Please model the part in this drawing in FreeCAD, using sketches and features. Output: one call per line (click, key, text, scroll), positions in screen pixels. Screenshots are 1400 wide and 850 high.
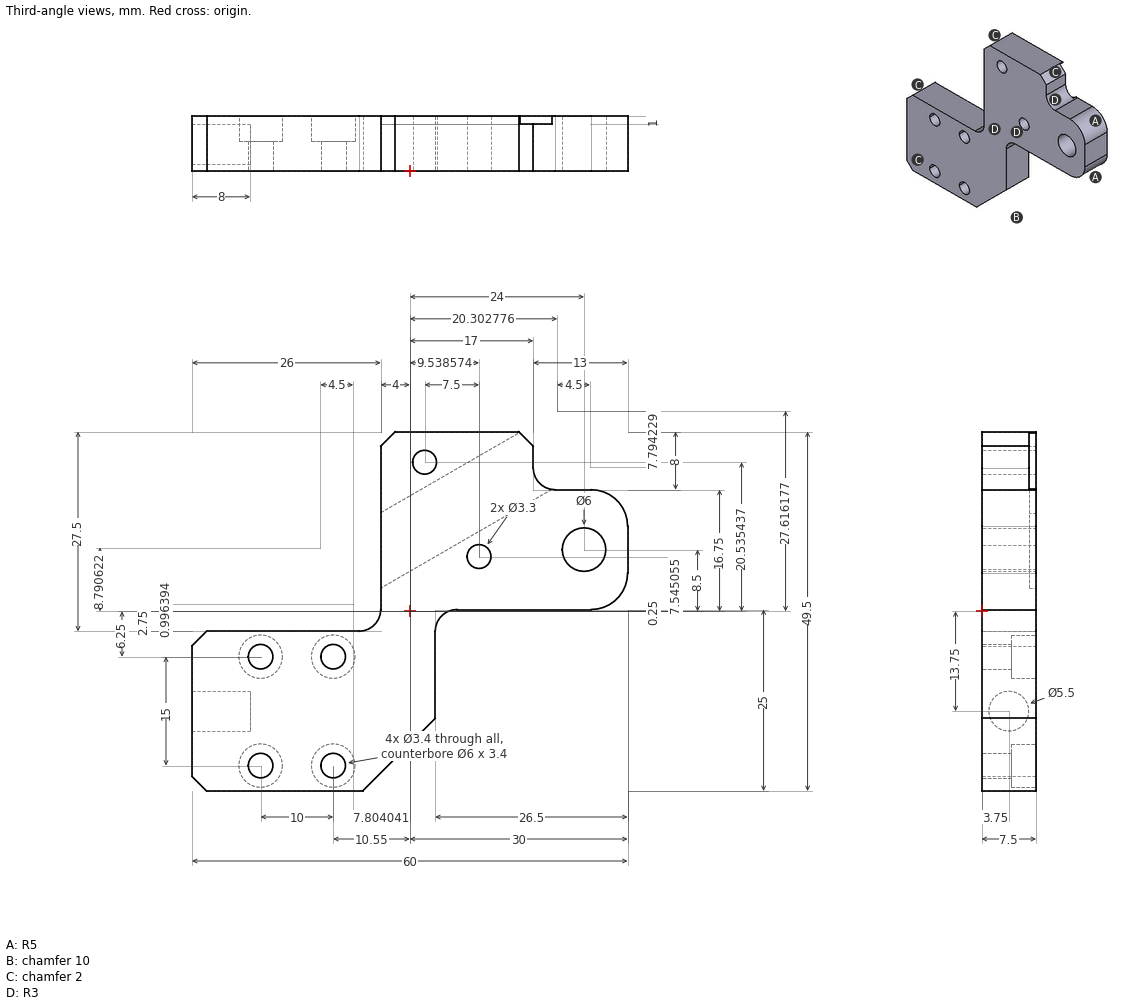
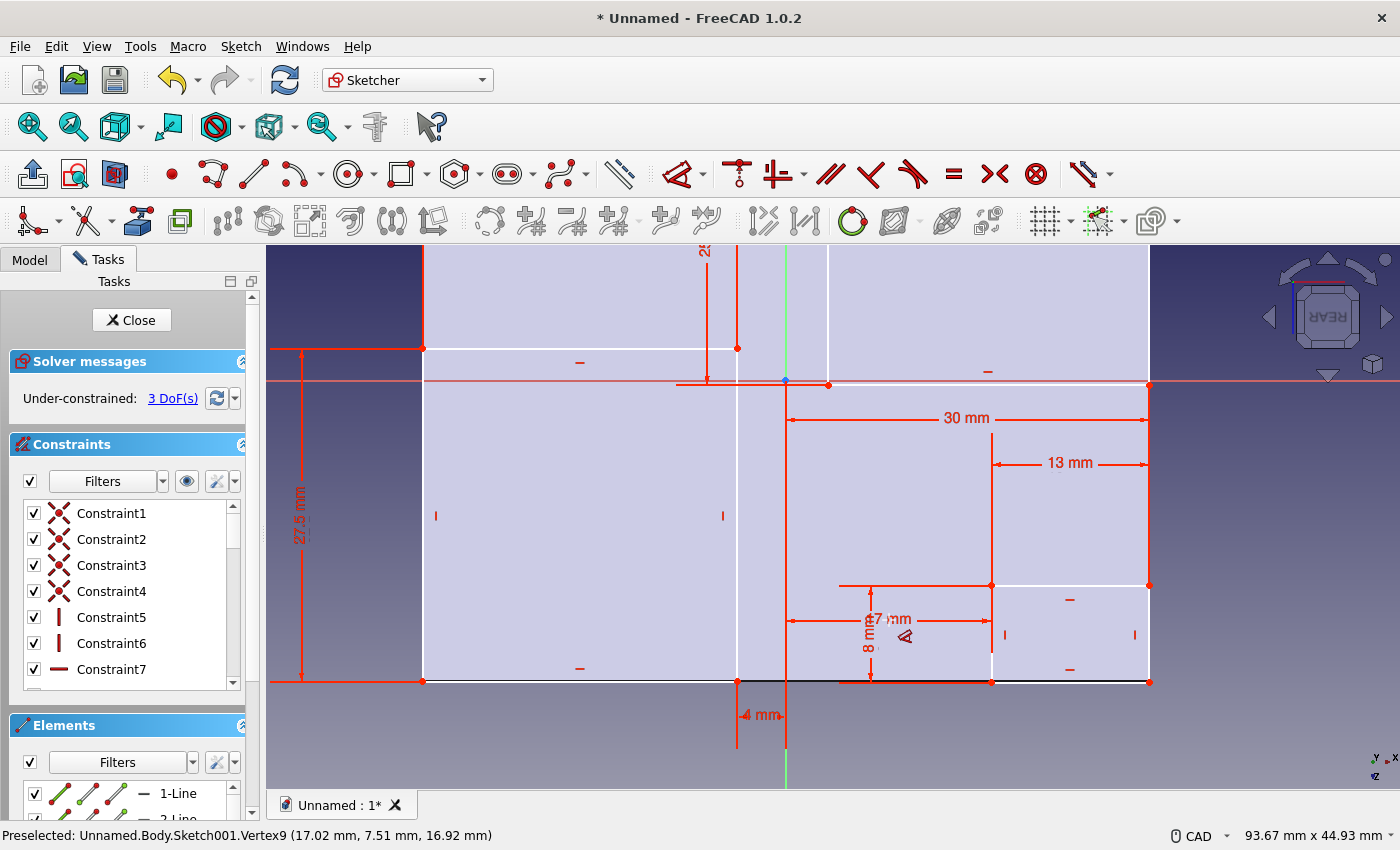
scroll(828, 385, up, 13)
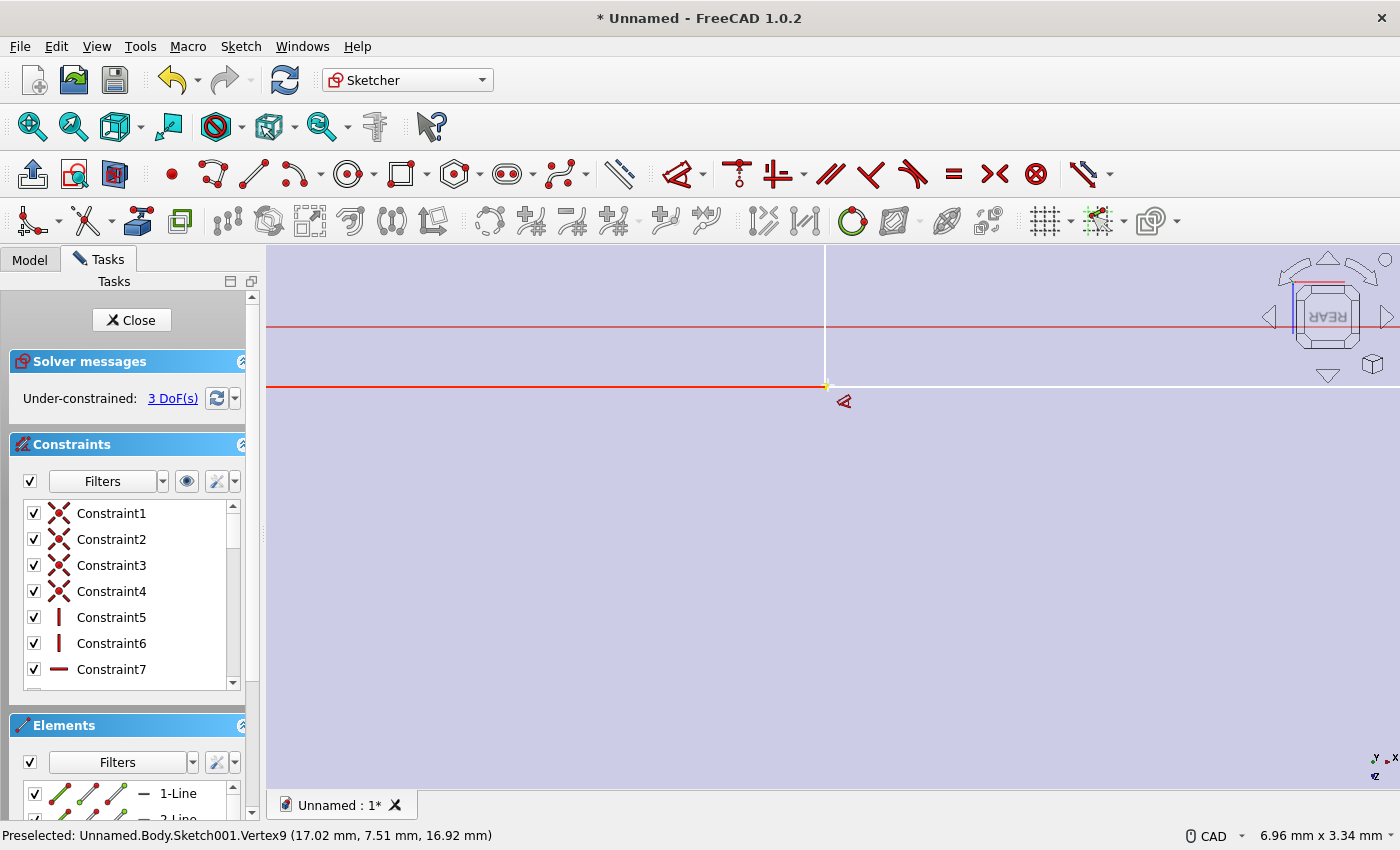
click(825, 387)
click(859, 357)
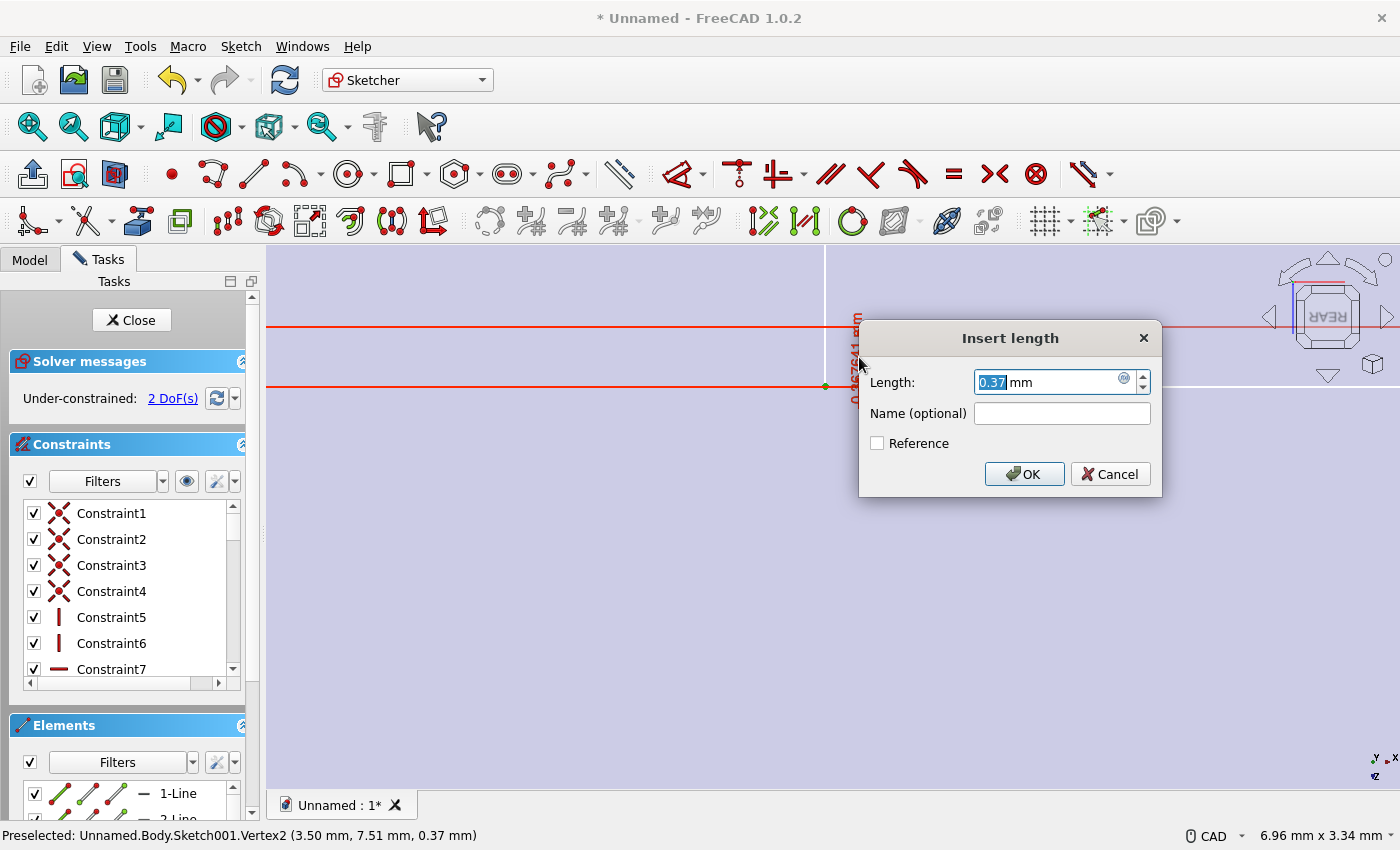
text(0.25)
key(Return)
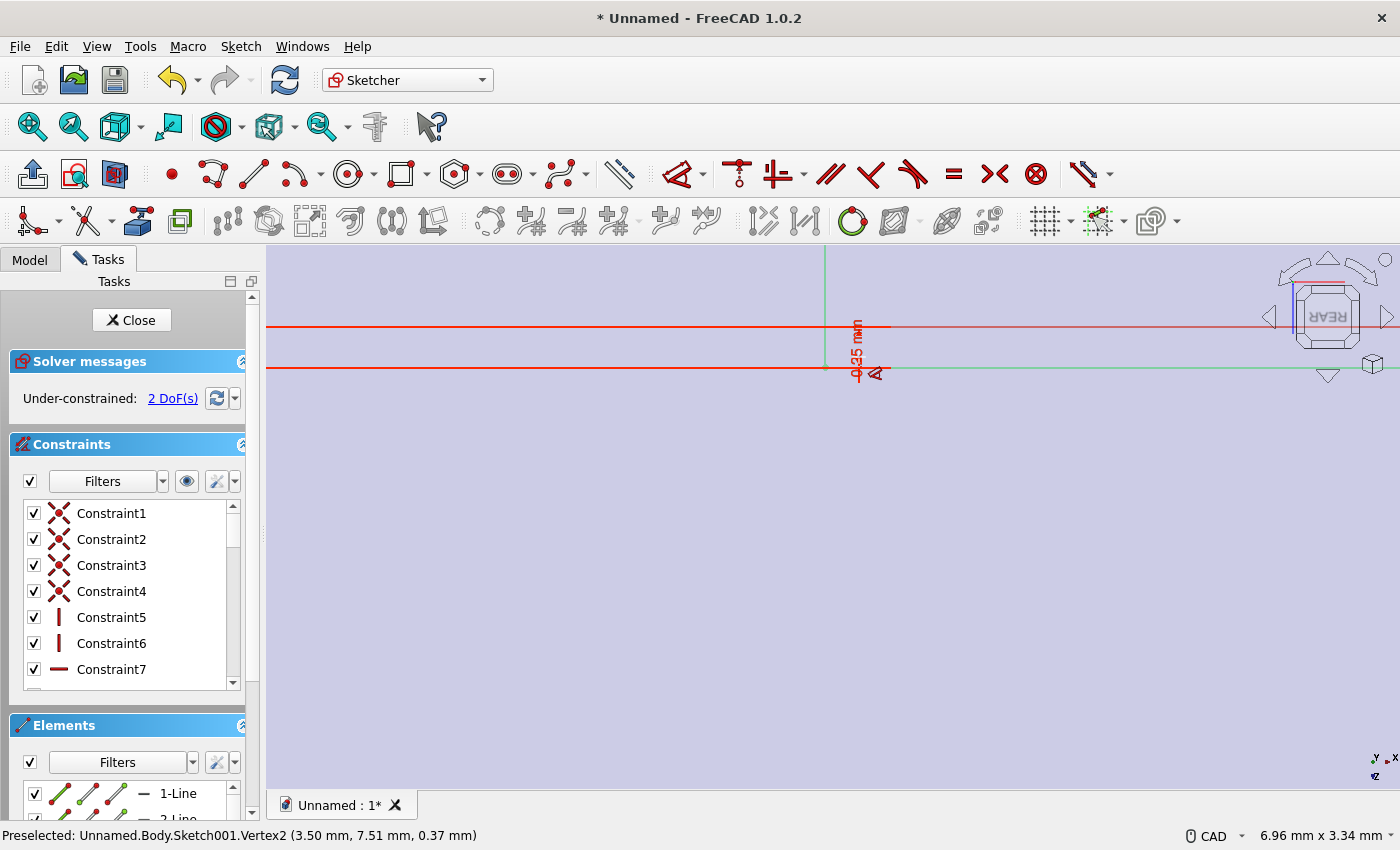
scroll(791, 527, down, 15)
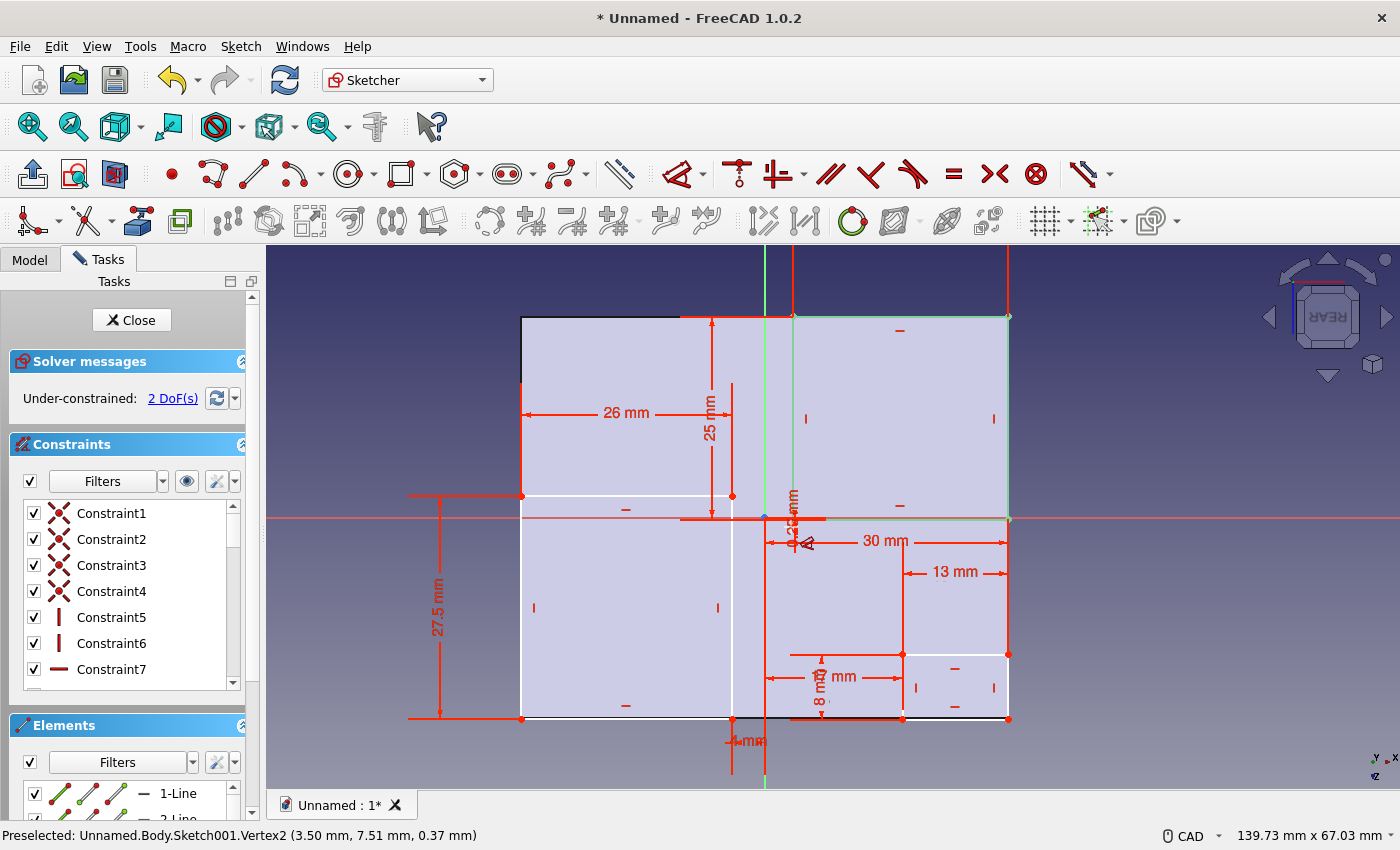
scroll(521, 496, up, 3)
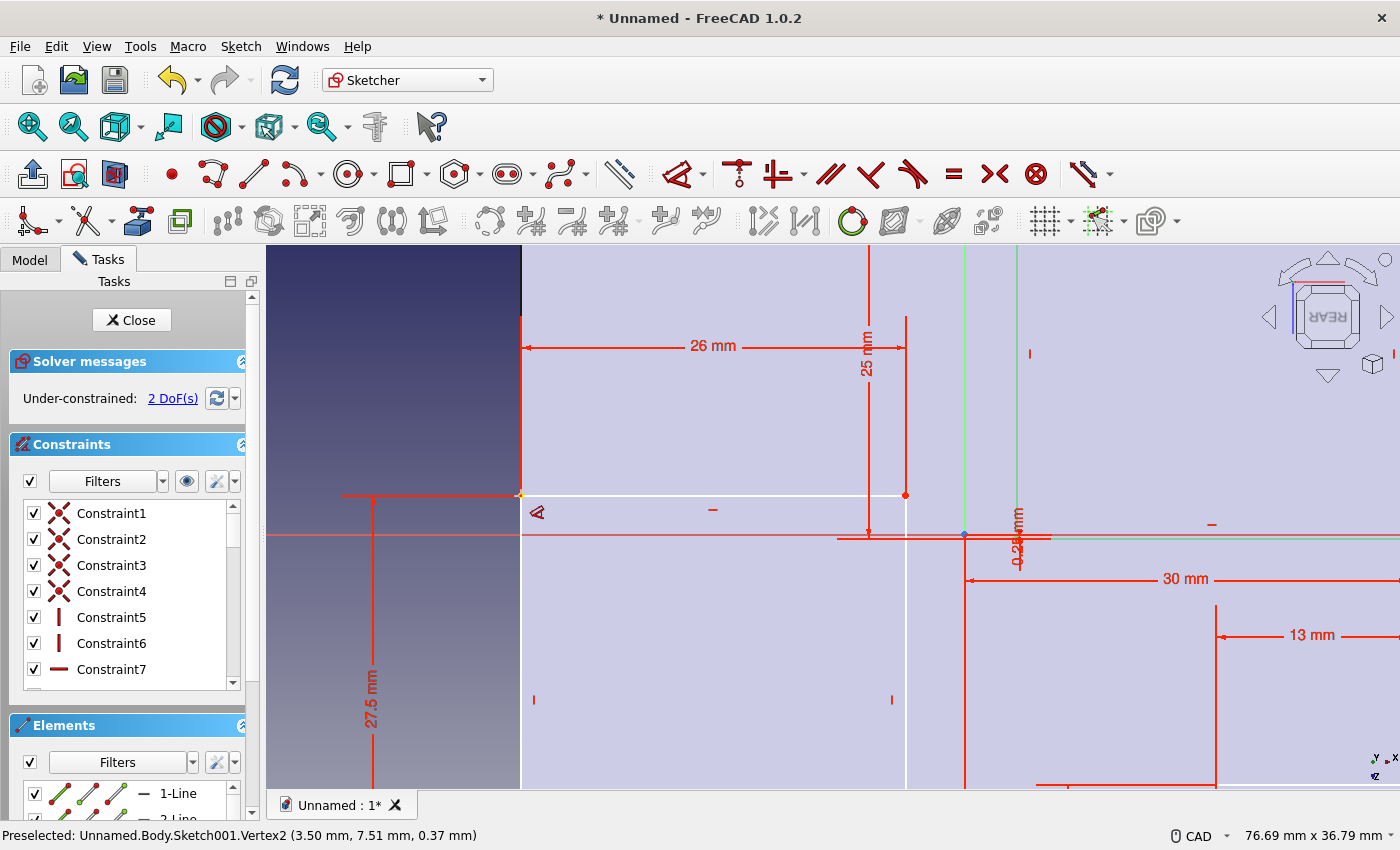
click(521, 496)
click(487, 515)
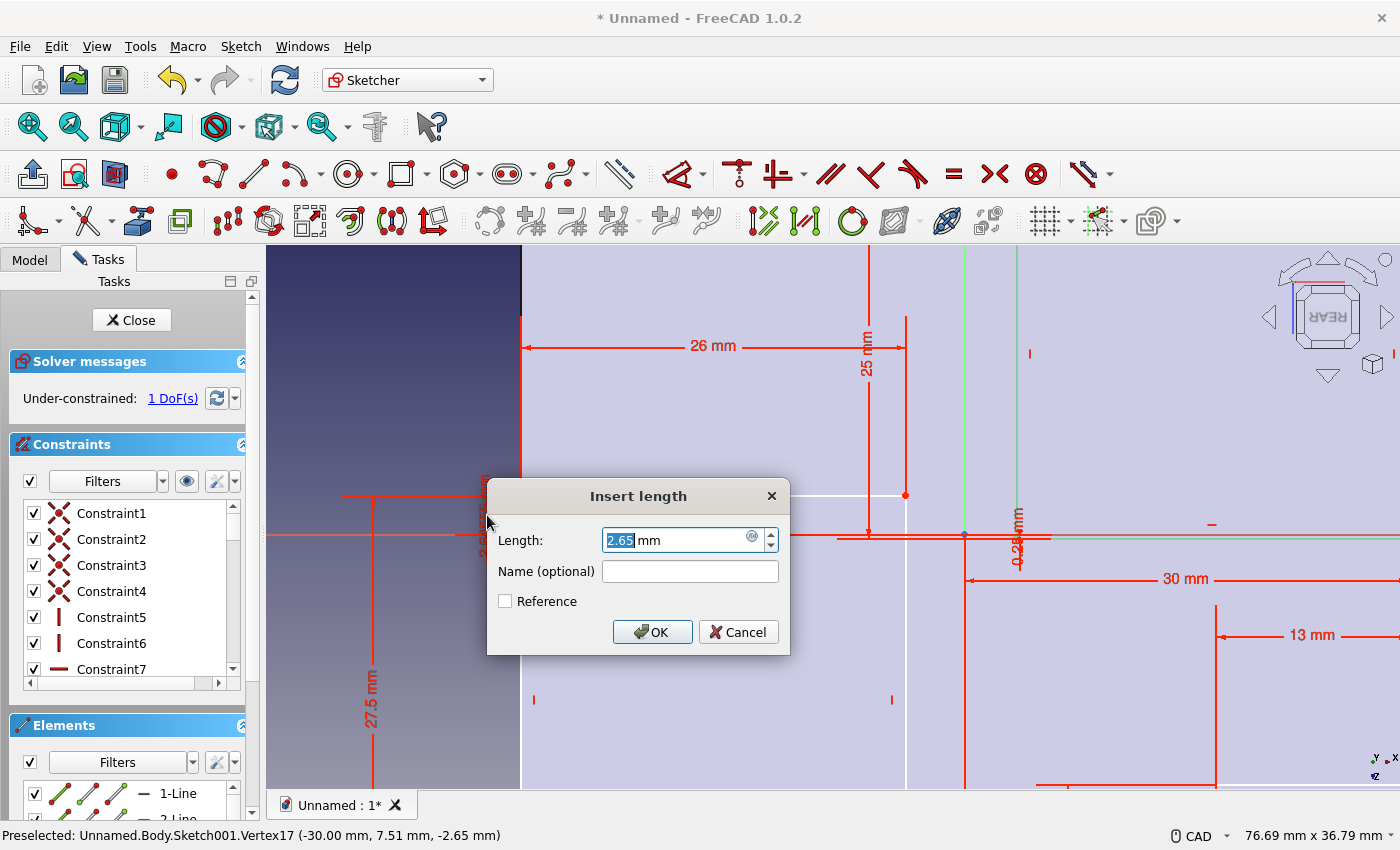
text(2.75)
key(Return)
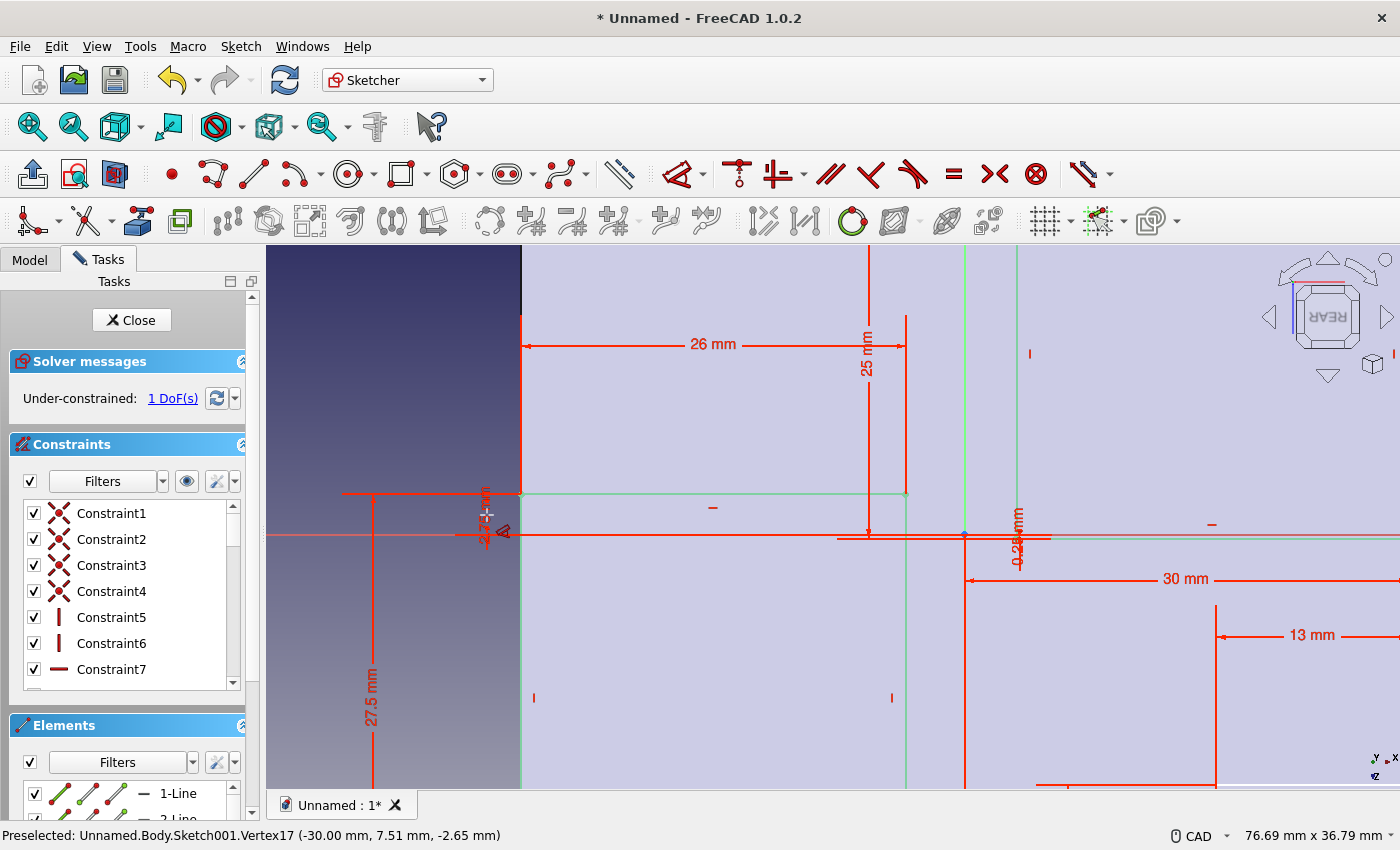
scroll(601, 502, down, 4)